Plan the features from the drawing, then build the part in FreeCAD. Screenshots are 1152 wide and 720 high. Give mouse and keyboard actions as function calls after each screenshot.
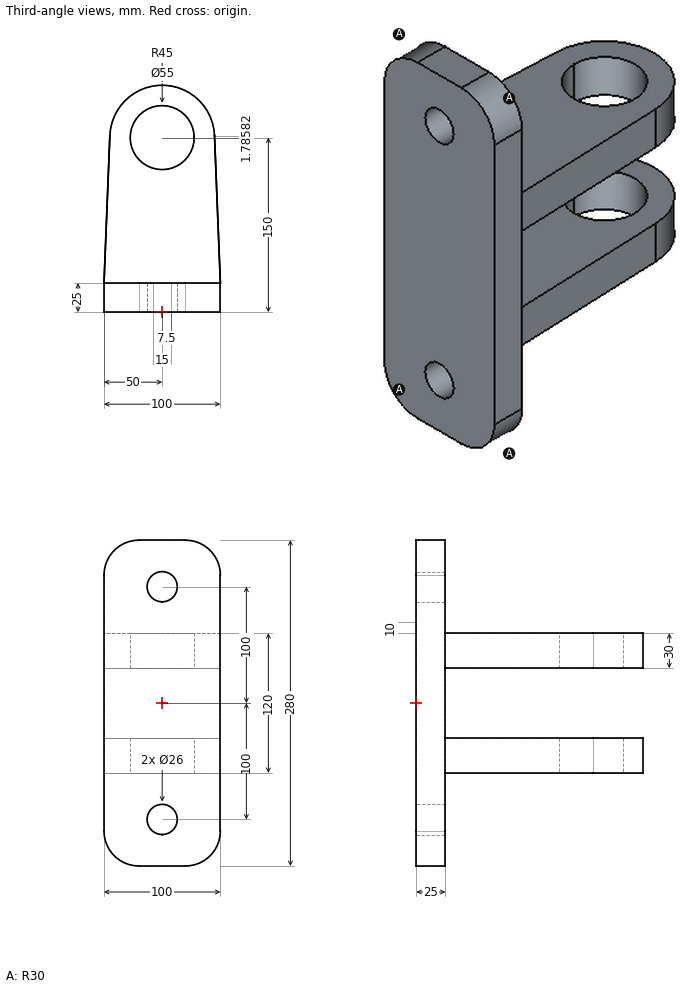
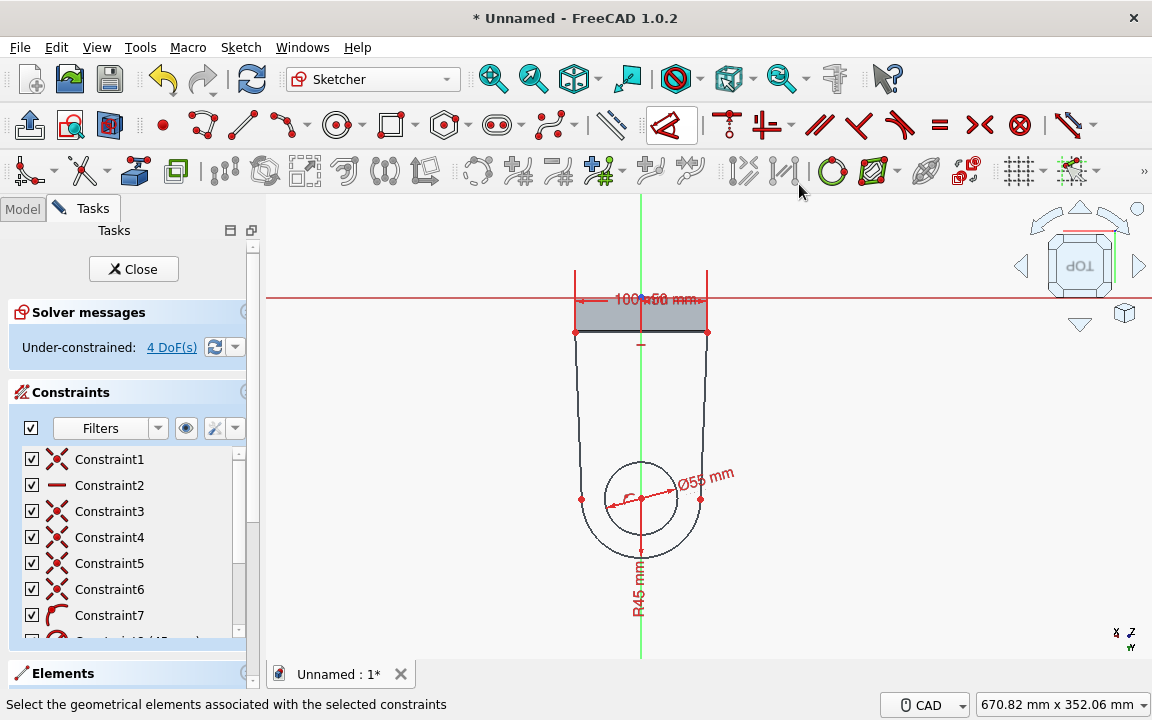
click(707, 332)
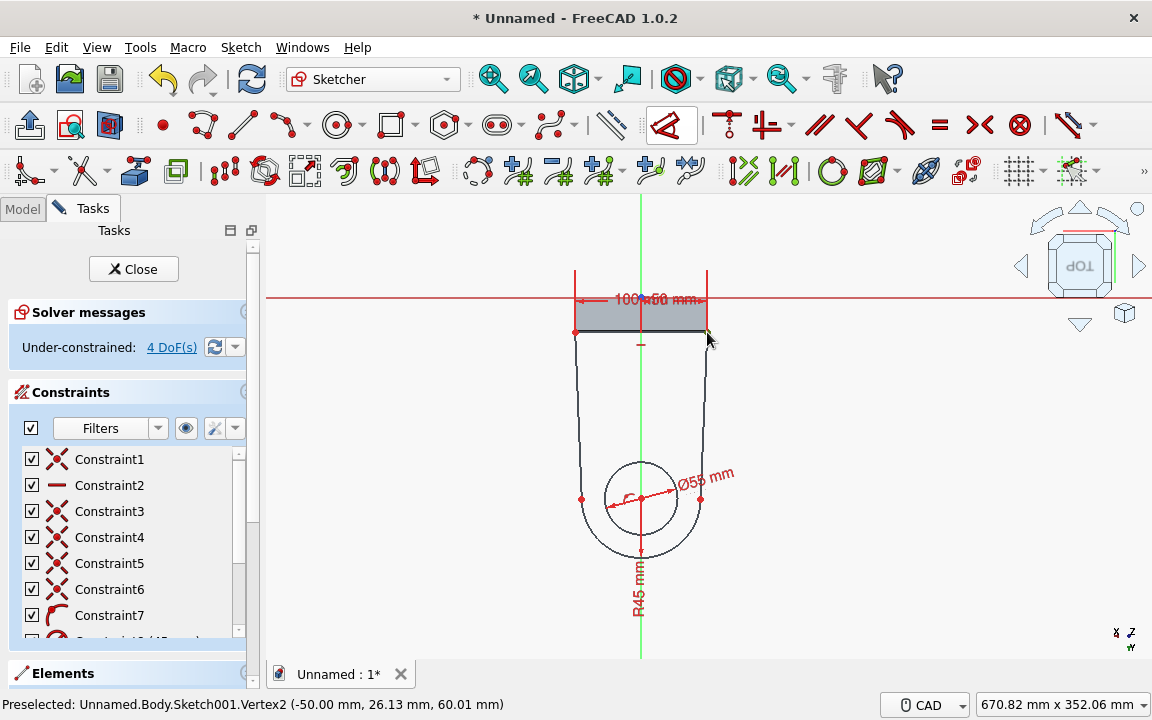
key(i)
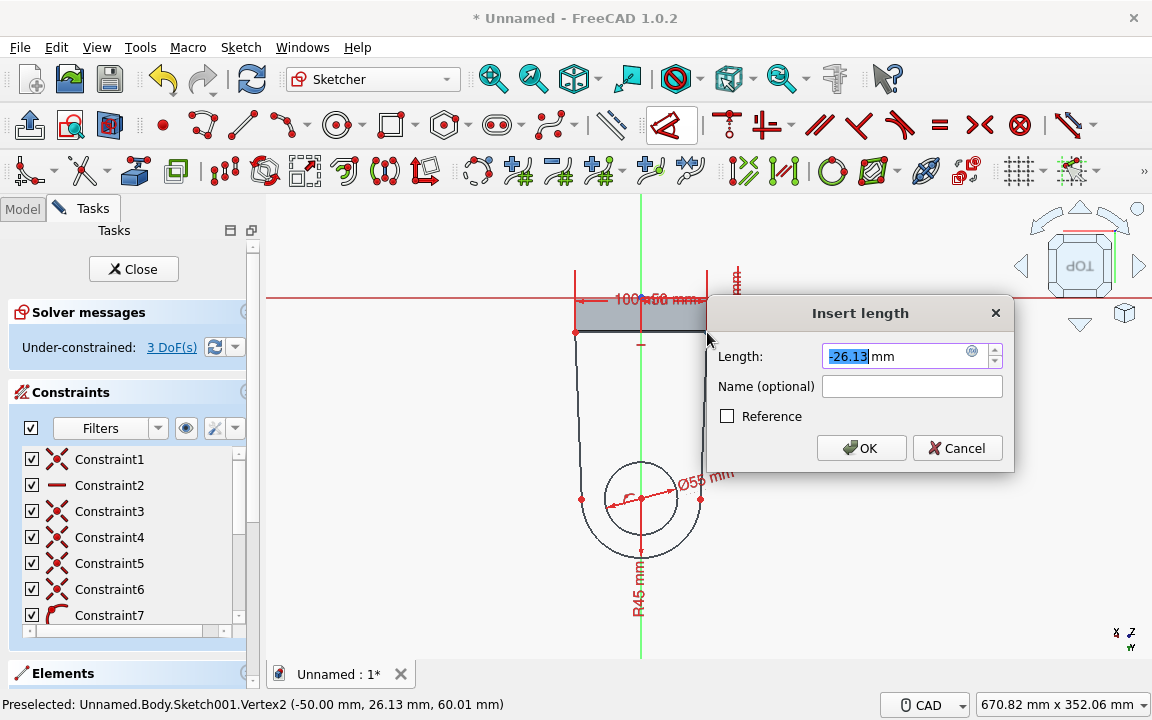
text(-25)
key(Return)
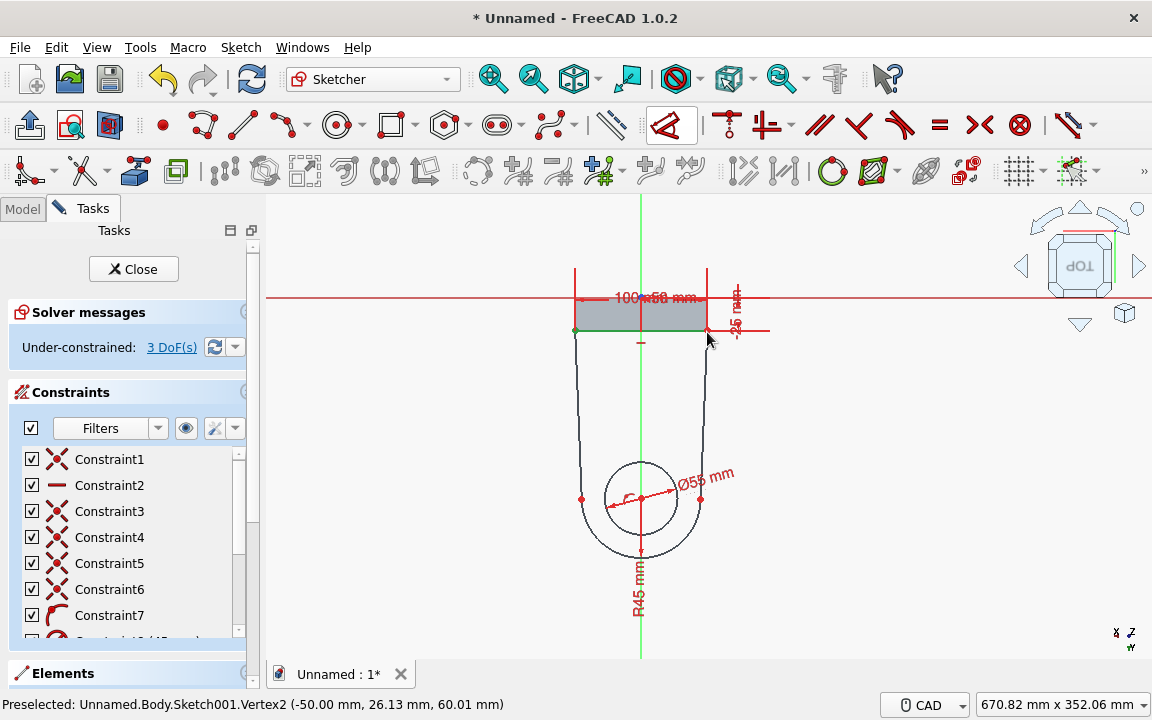
click(641, 499)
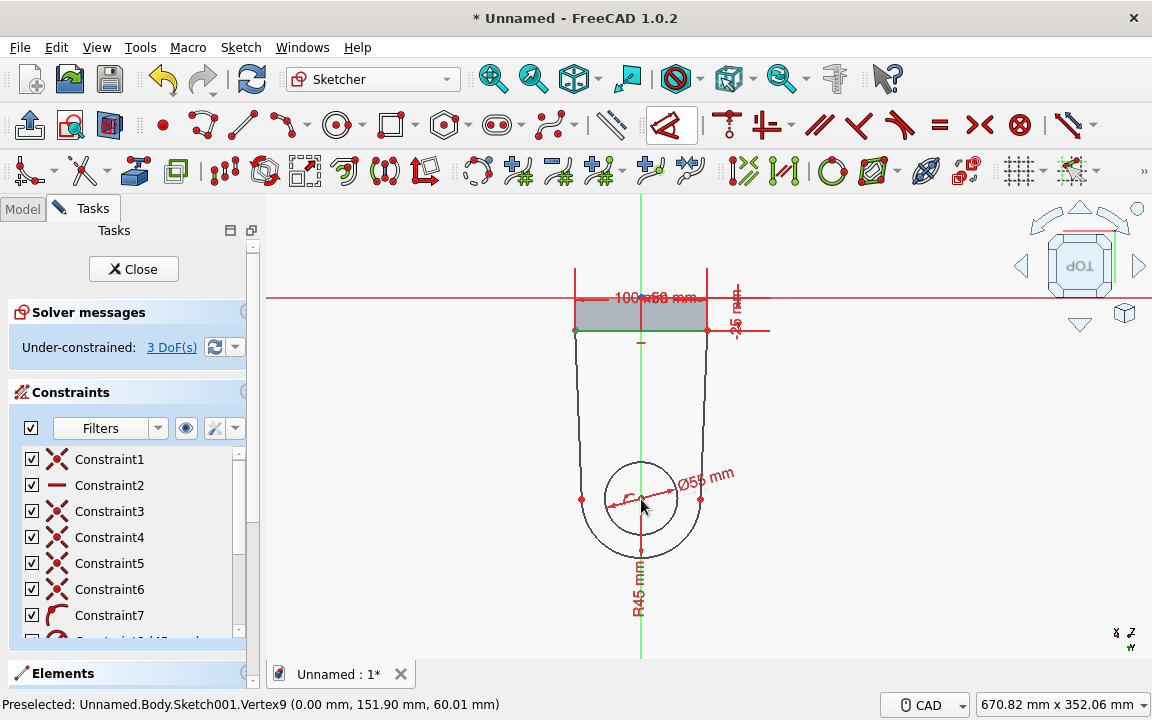
click(692, 126)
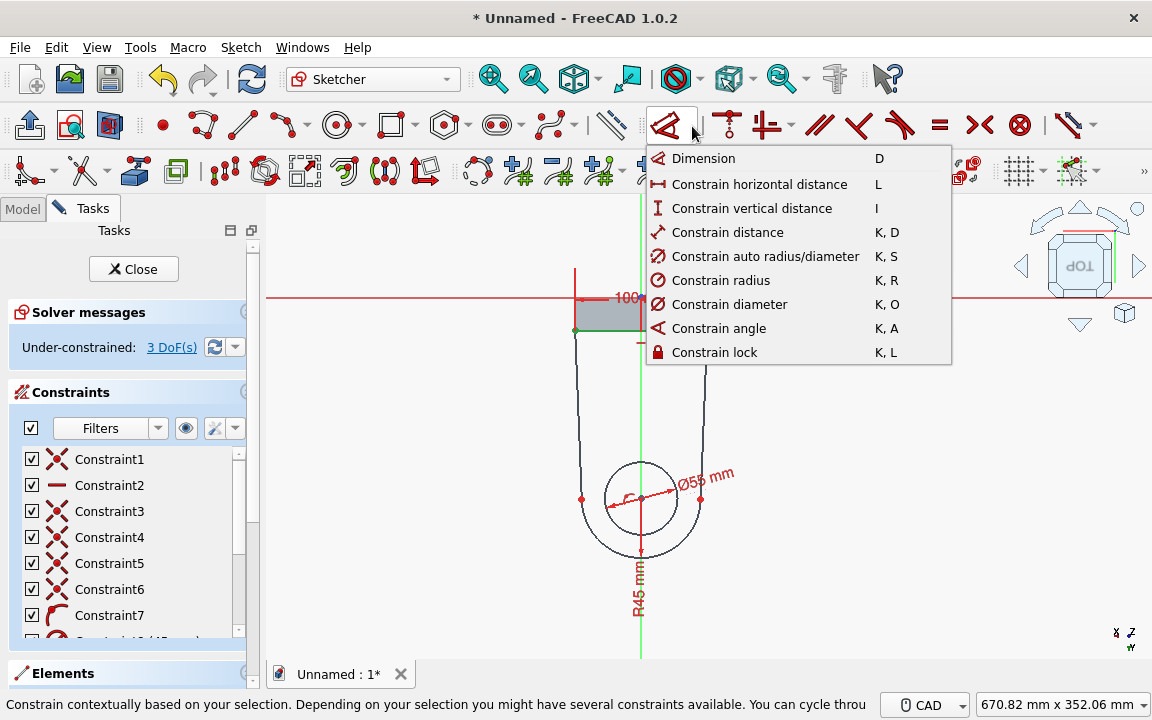
click(799, 208)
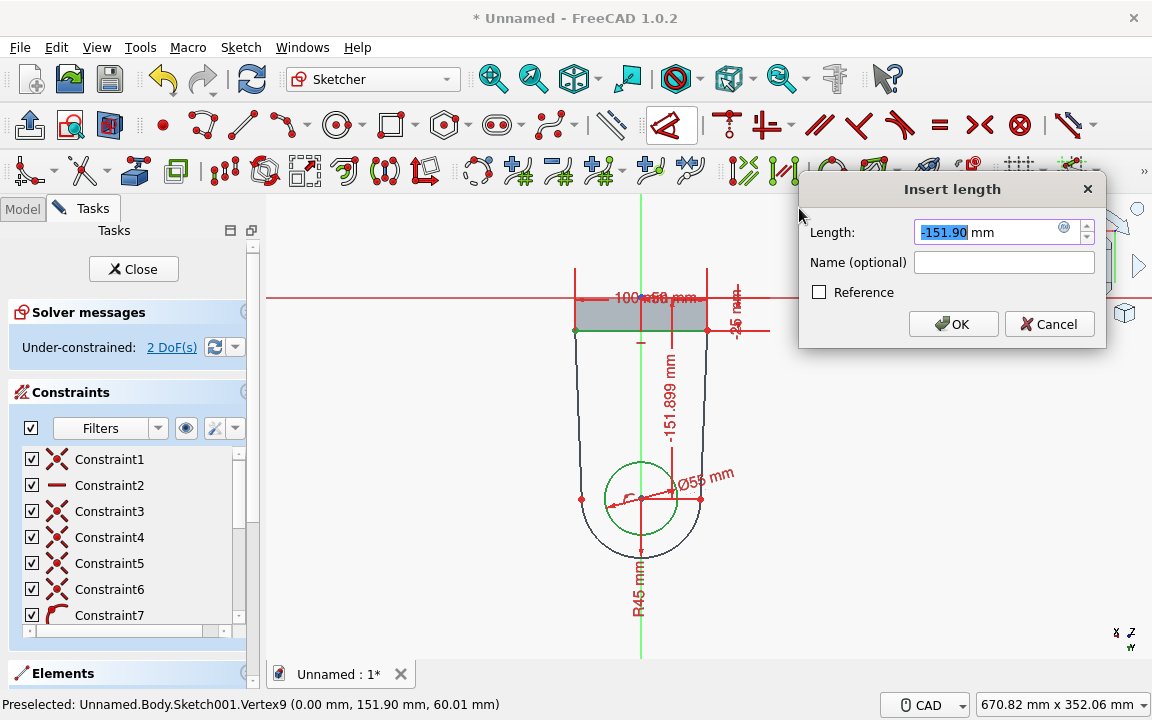
text(-150)
key(Return)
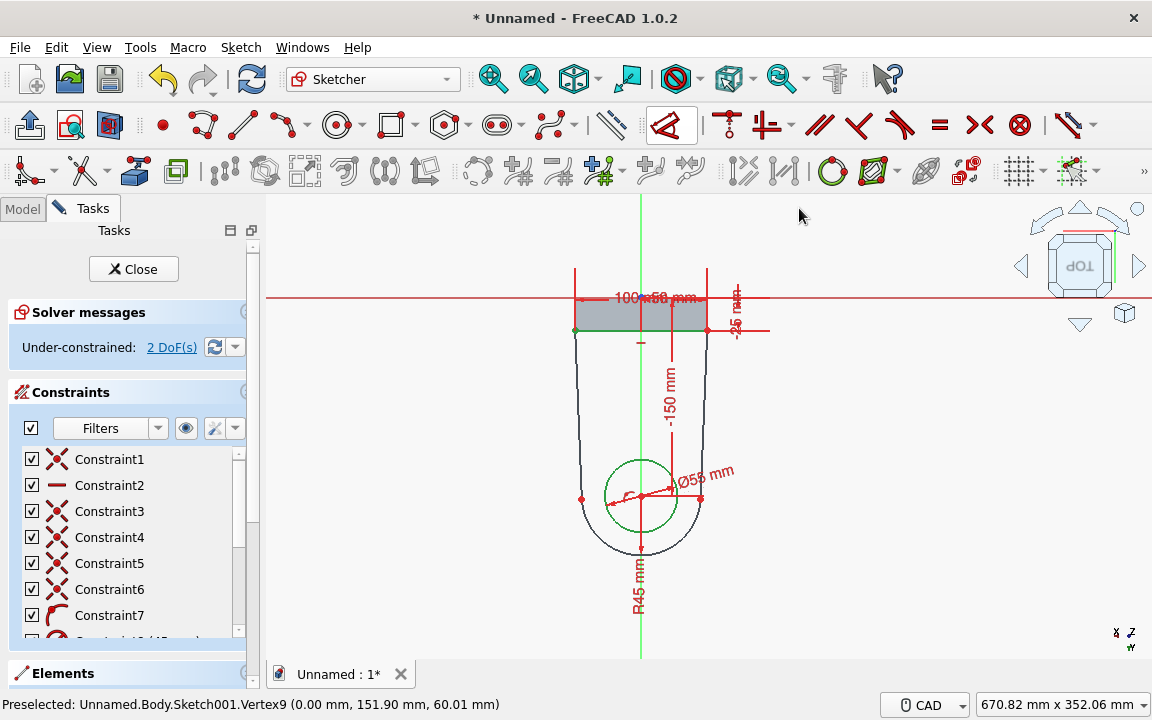
scroll(582, 500, up, 15)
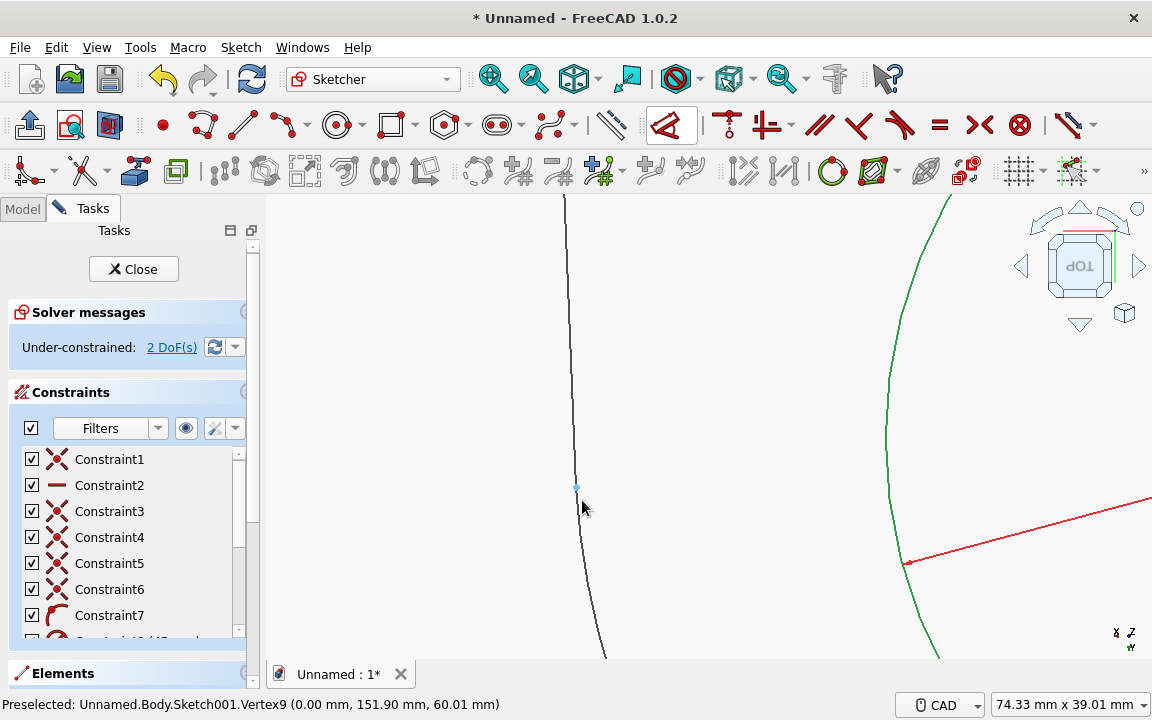
click(573, 481)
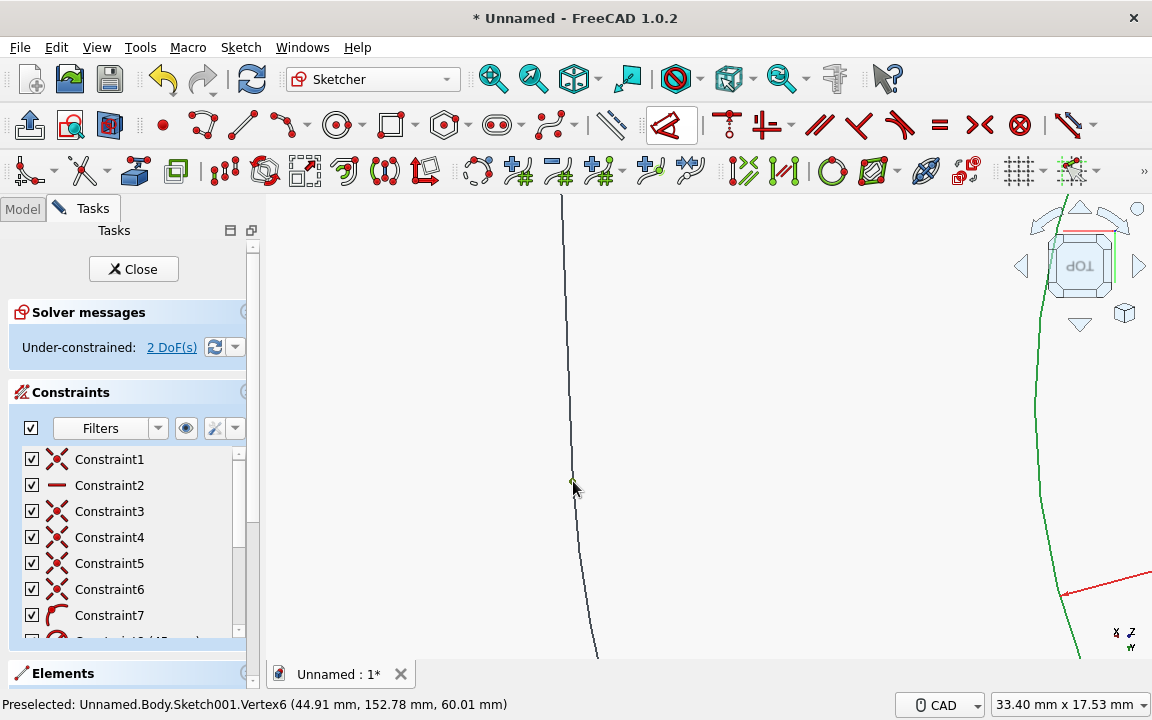
scroll(568, 518, down, 14)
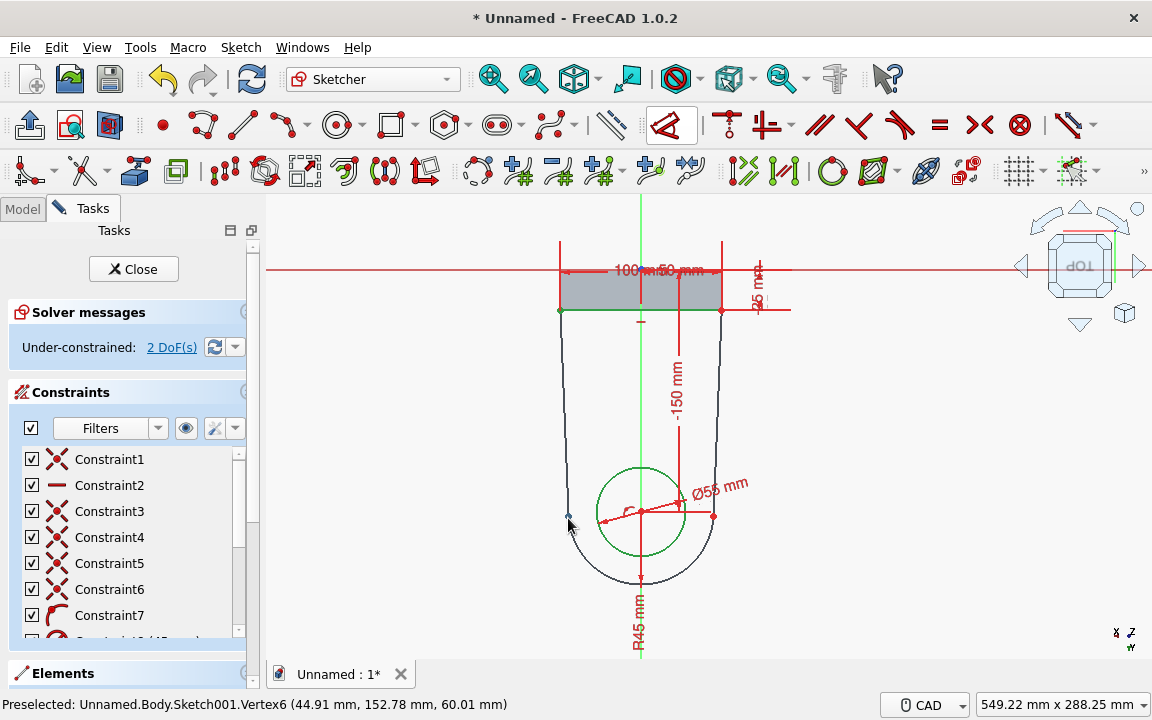
scroll(641, 512, up, 14)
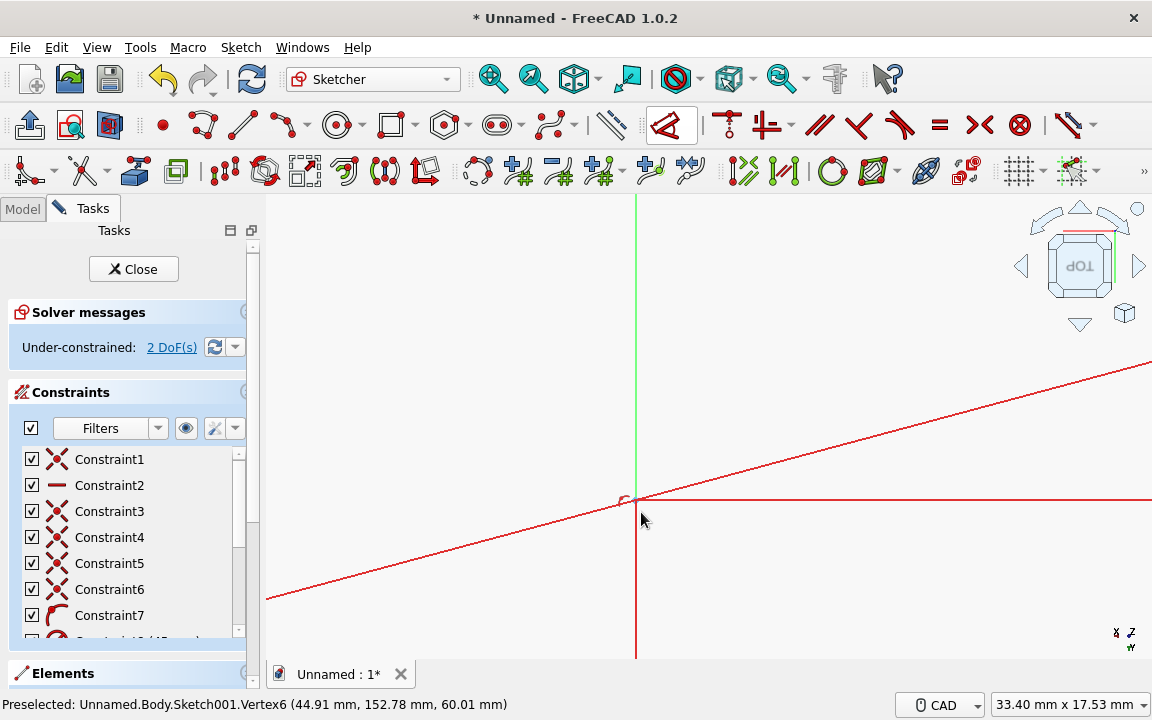
click(636, 500)